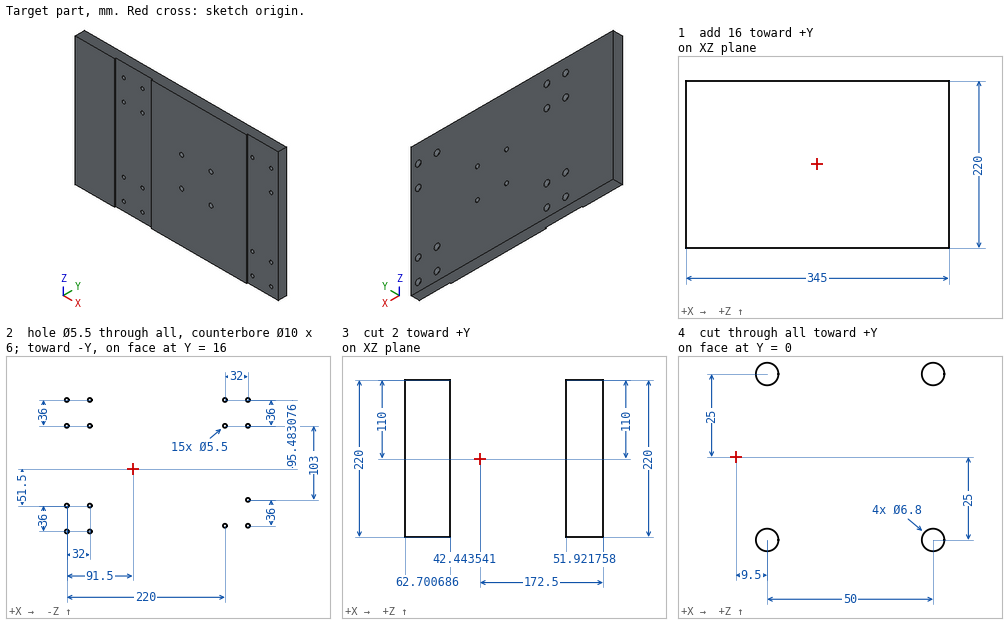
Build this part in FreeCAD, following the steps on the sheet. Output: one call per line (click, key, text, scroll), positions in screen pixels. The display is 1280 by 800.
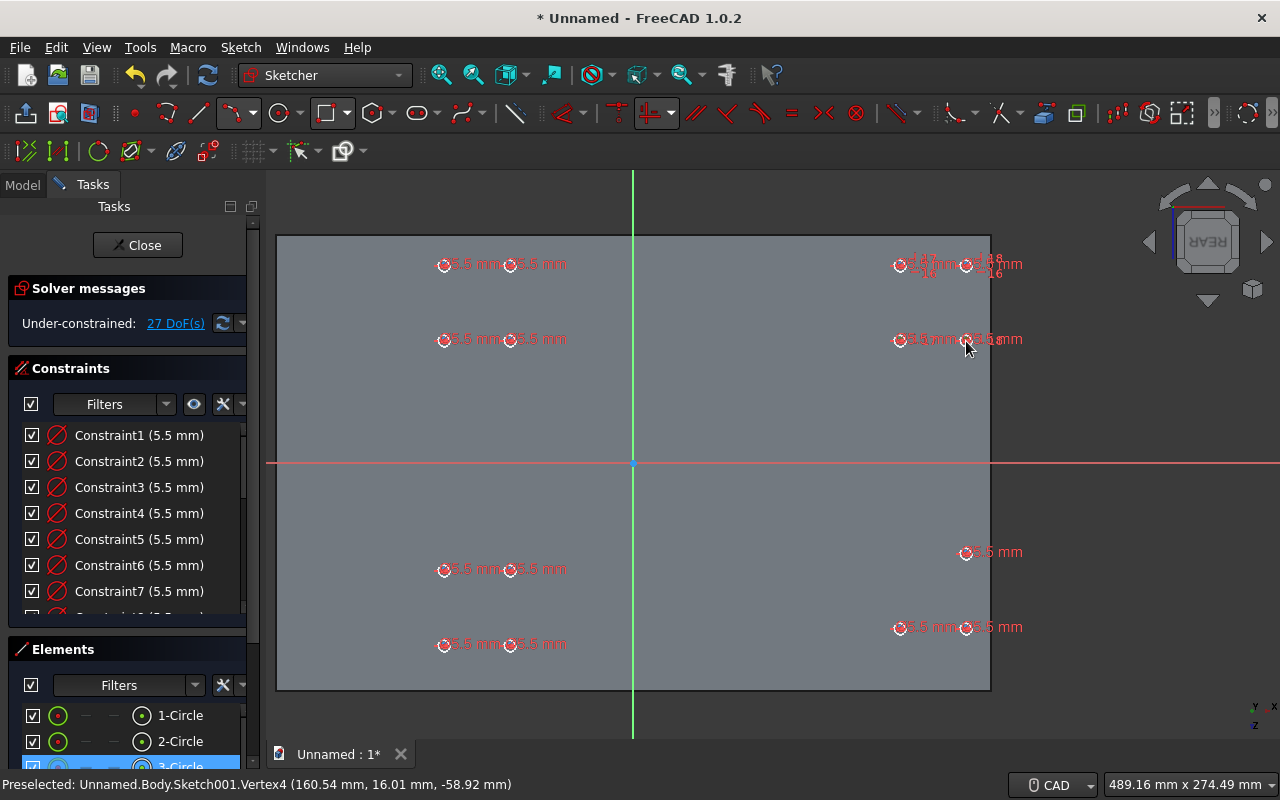
key(h)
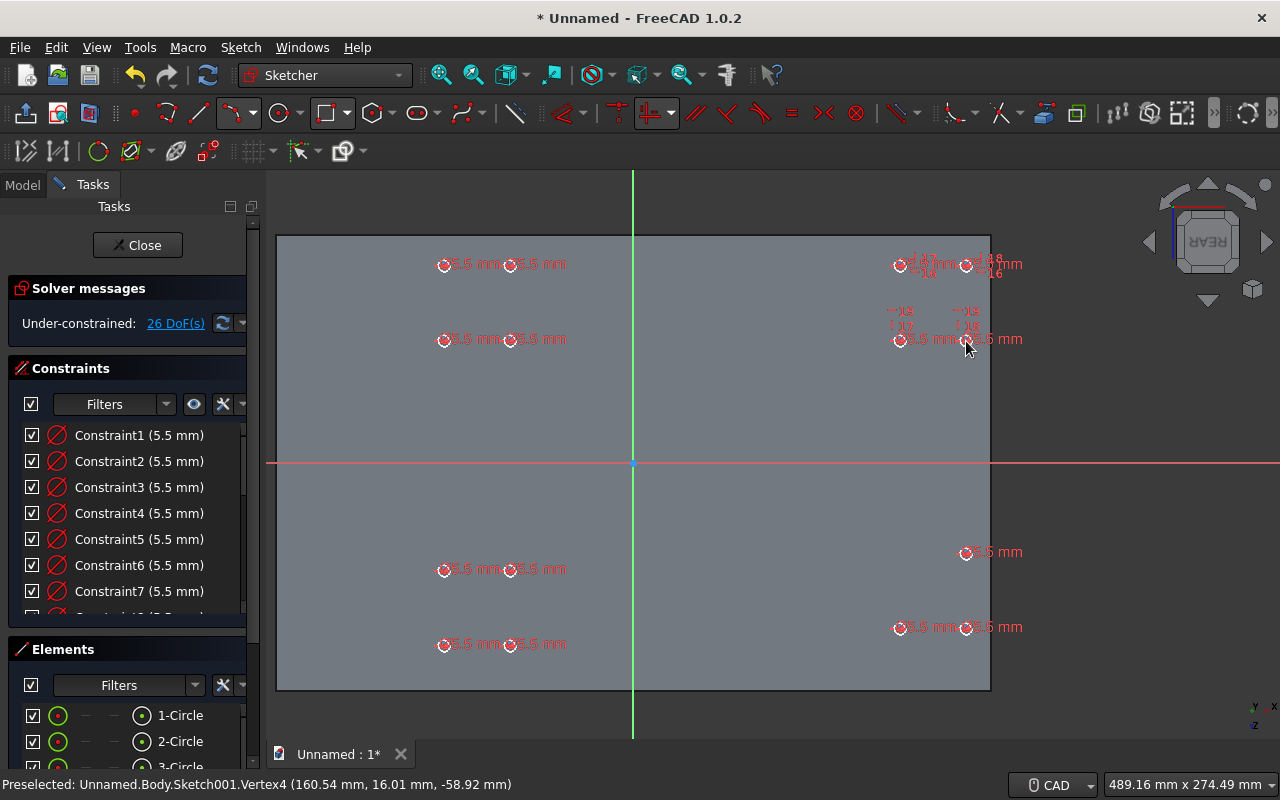
click(966, 341)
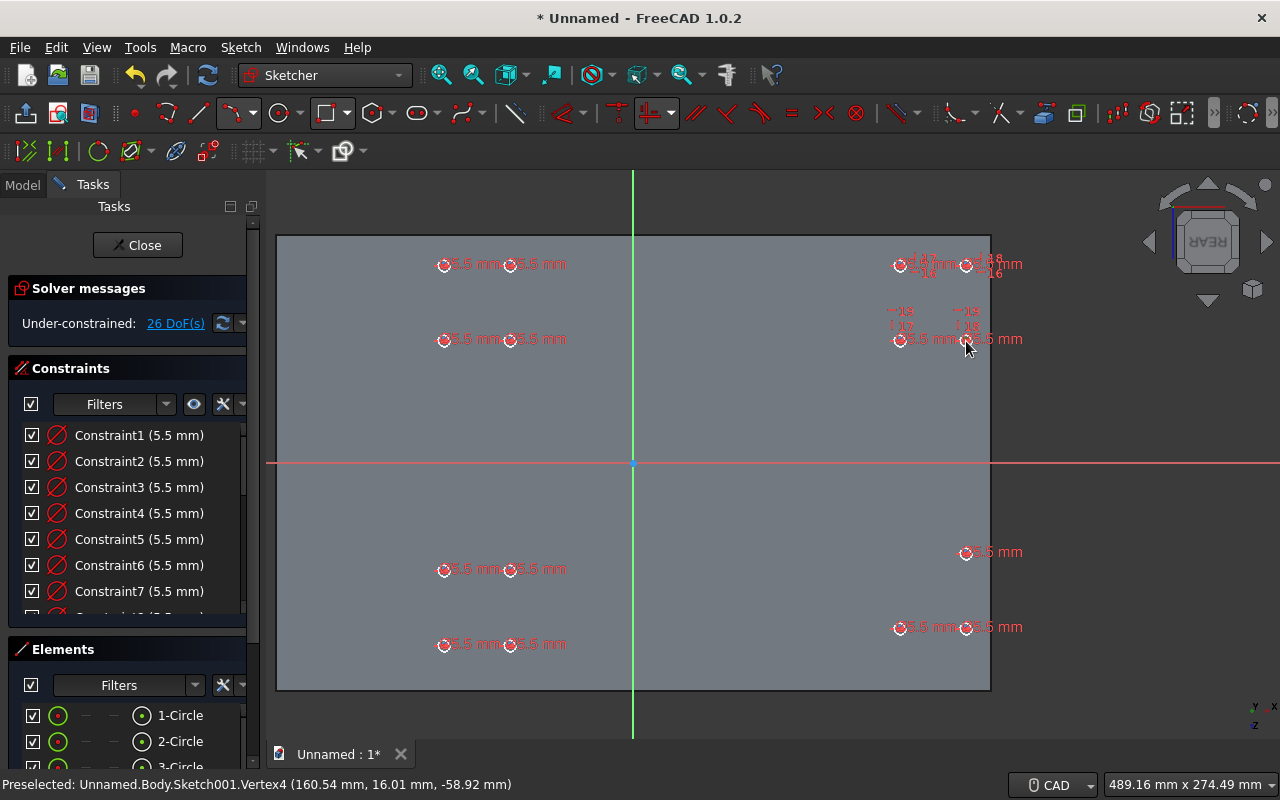
click(966, 554)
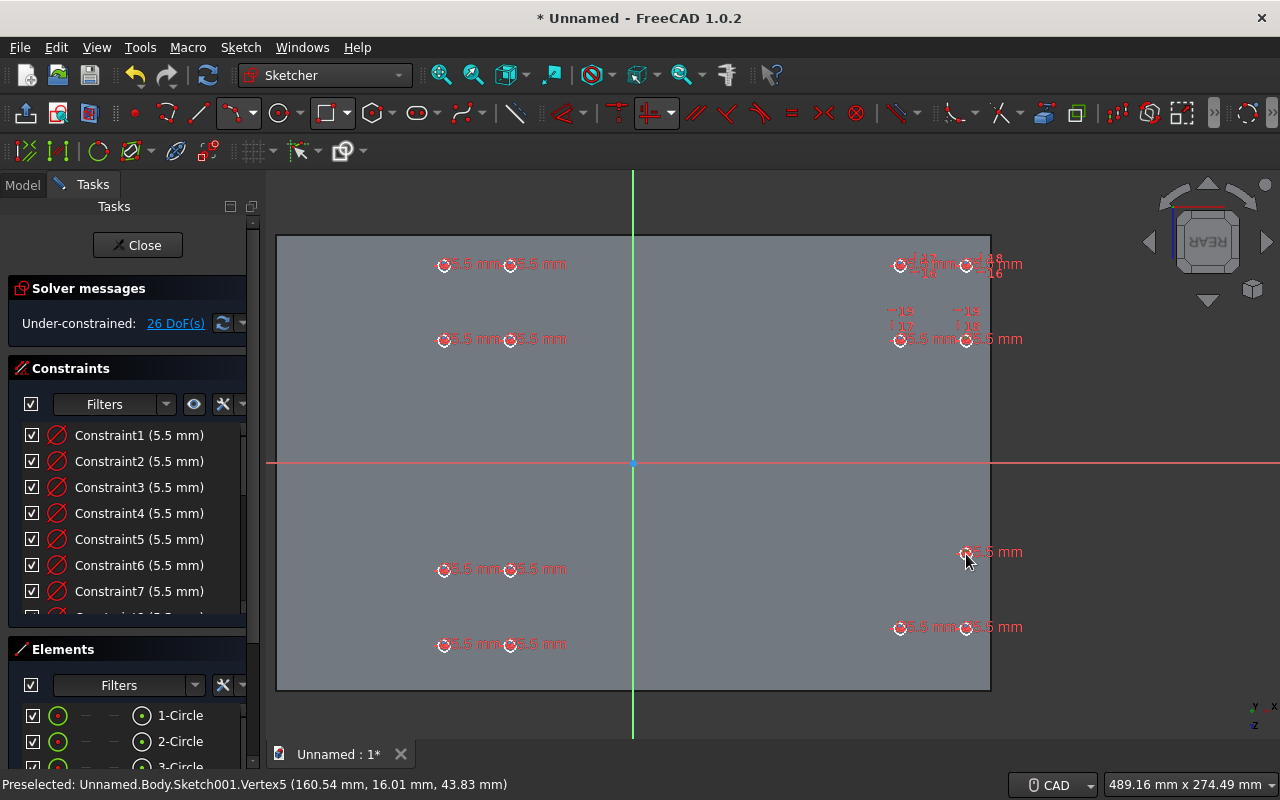
click(674, 114)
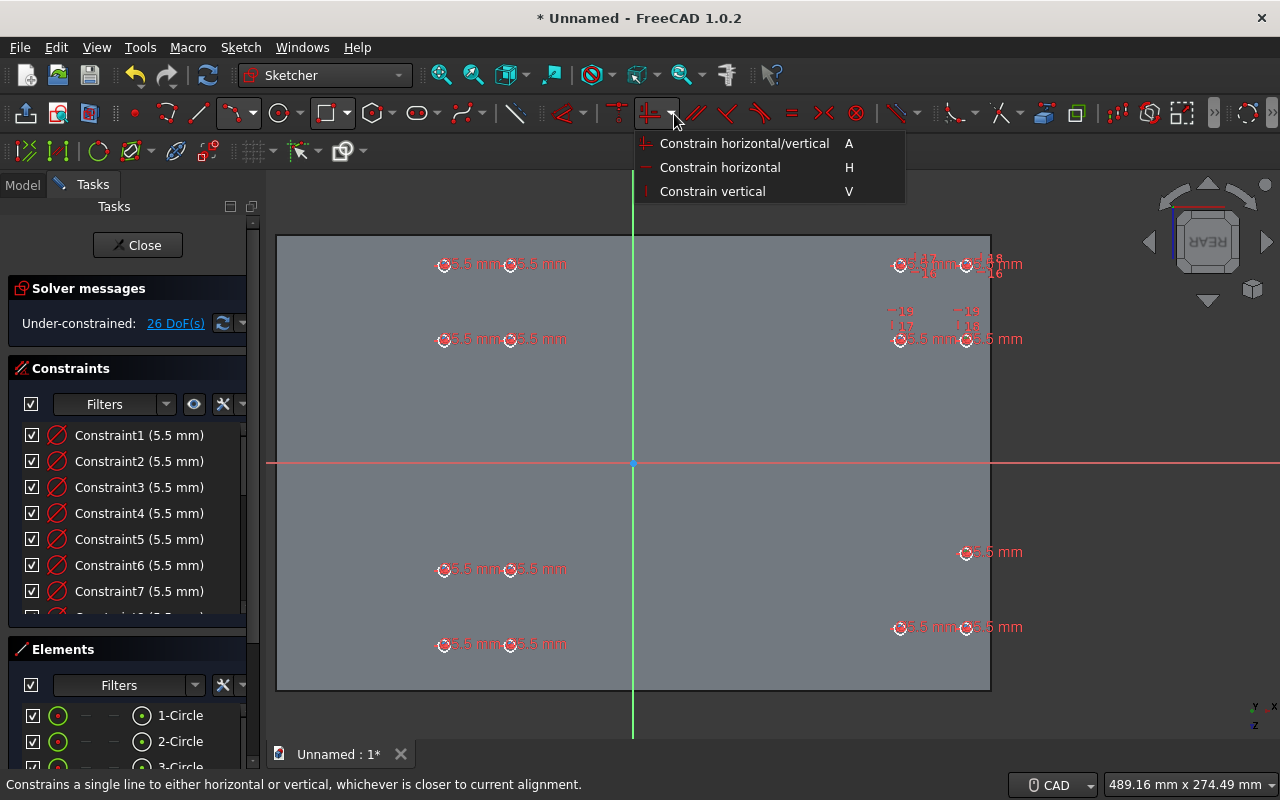
click(770, 191)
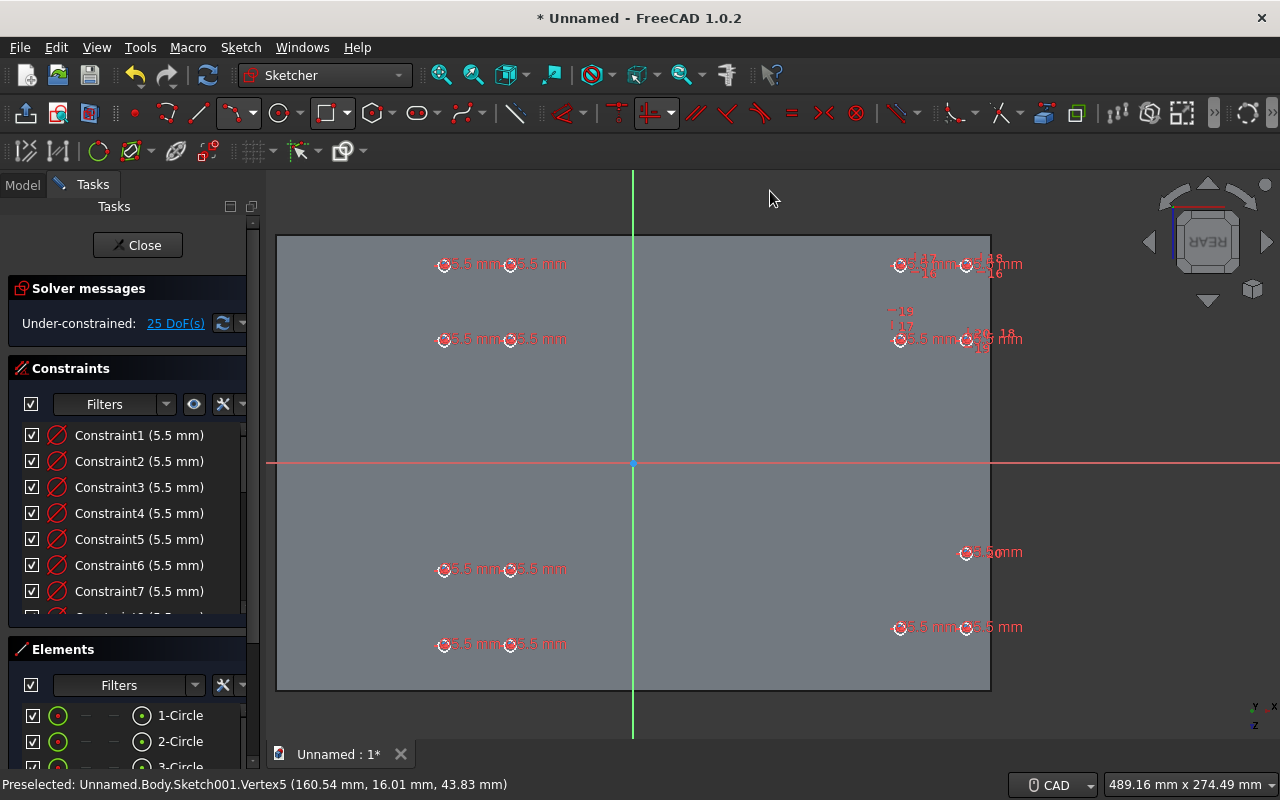
click(966, 554)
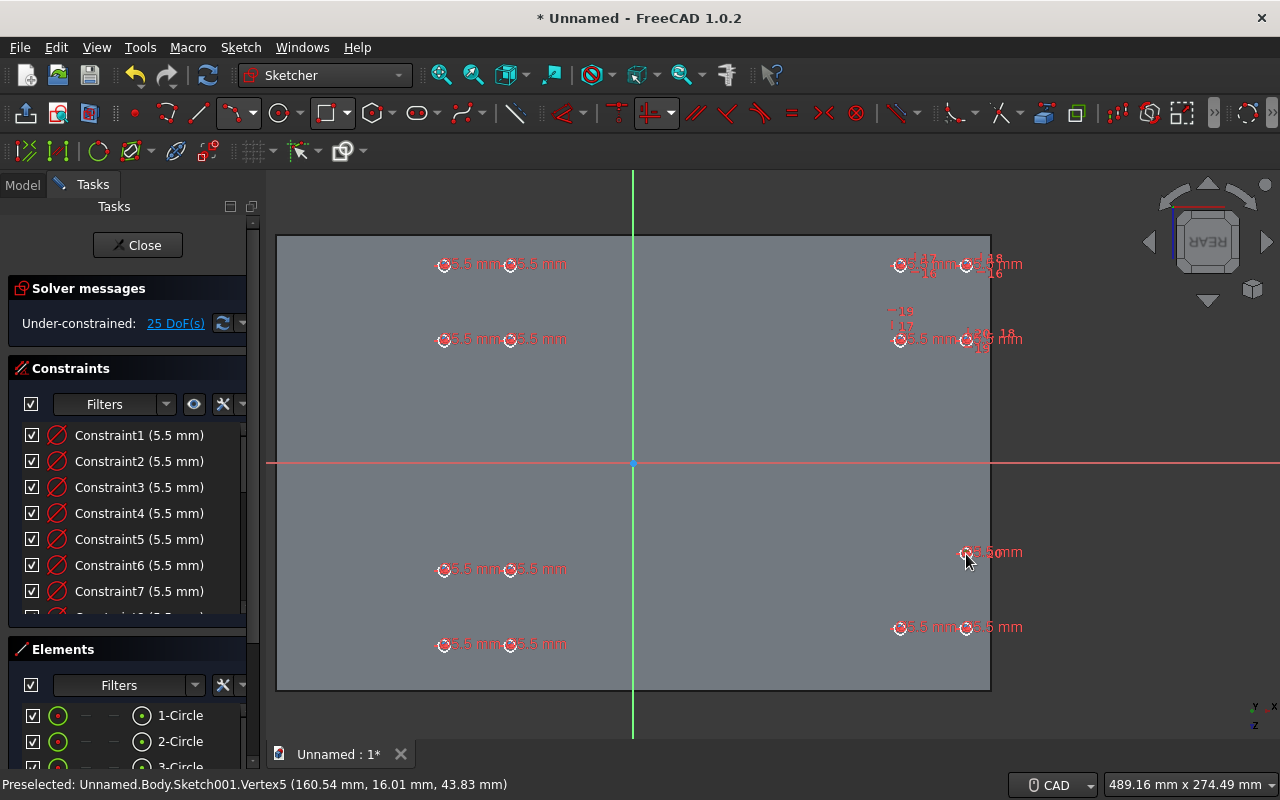
click(966, 629)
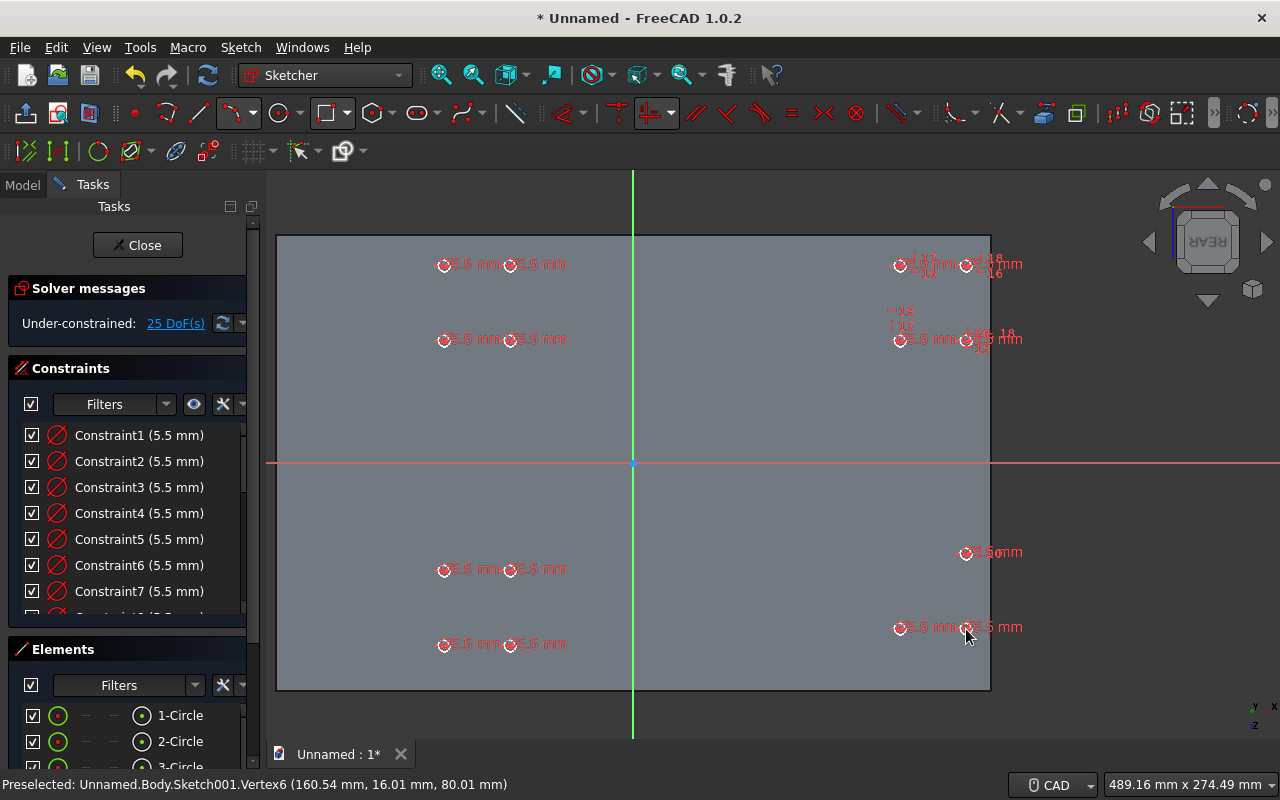
key(v)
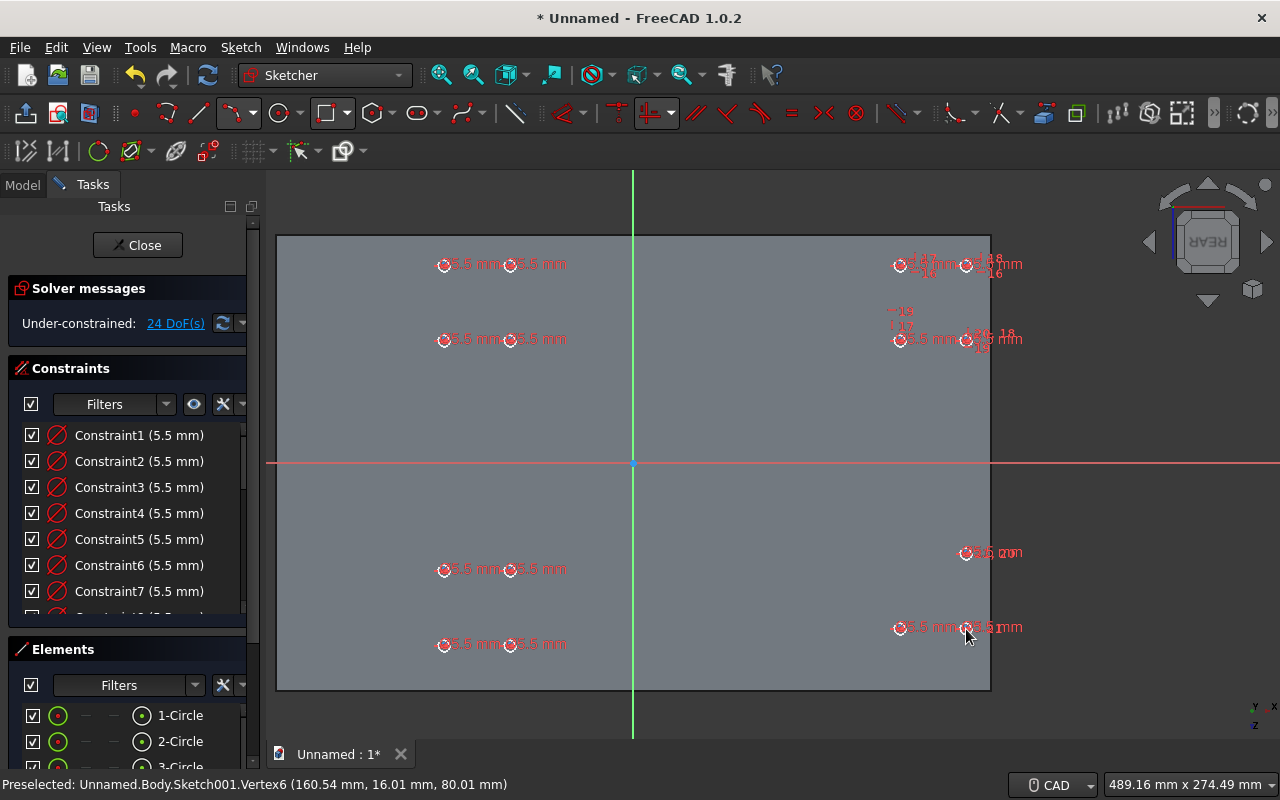
click(900, 341)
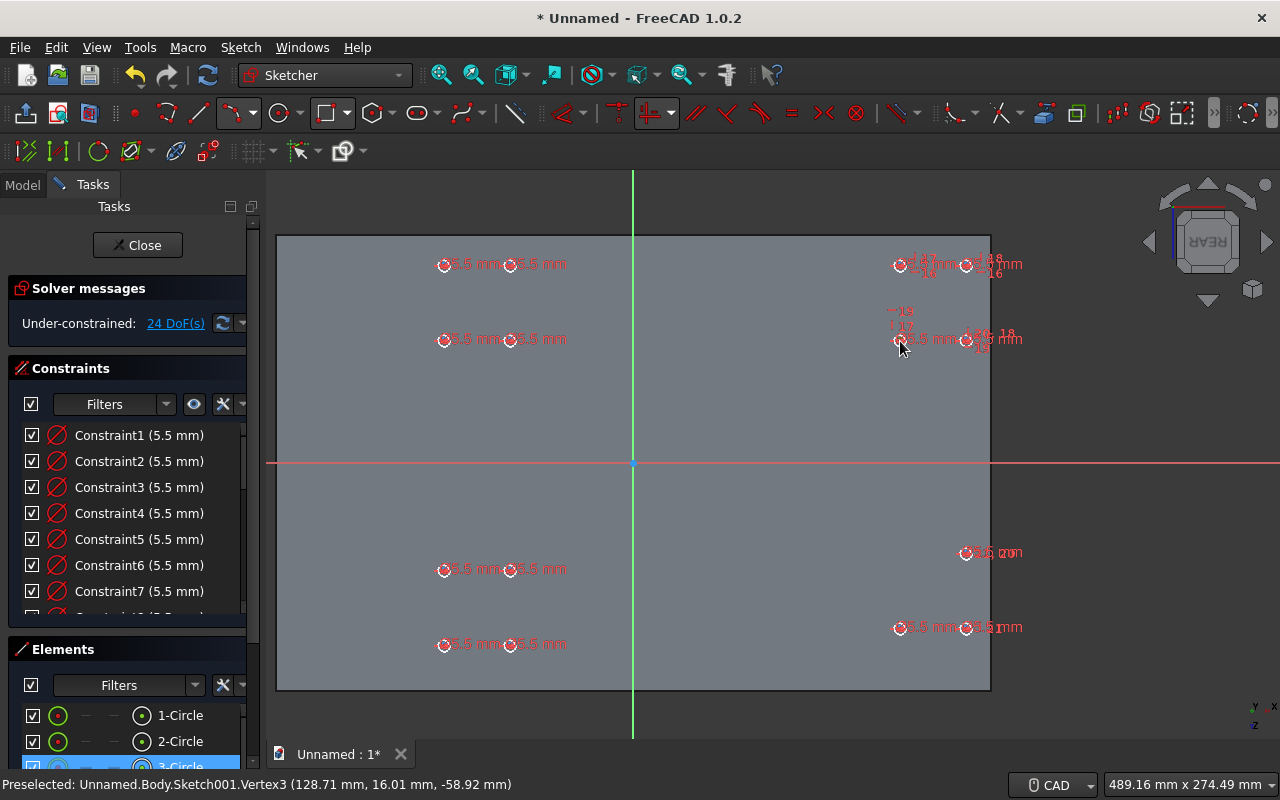
click(900, 629)